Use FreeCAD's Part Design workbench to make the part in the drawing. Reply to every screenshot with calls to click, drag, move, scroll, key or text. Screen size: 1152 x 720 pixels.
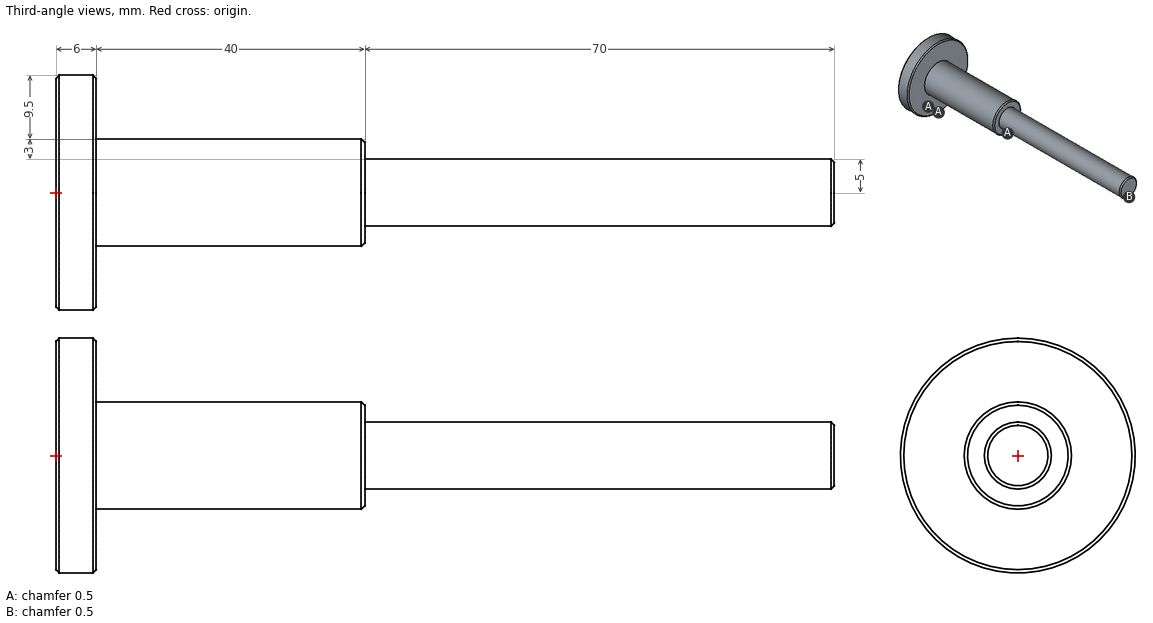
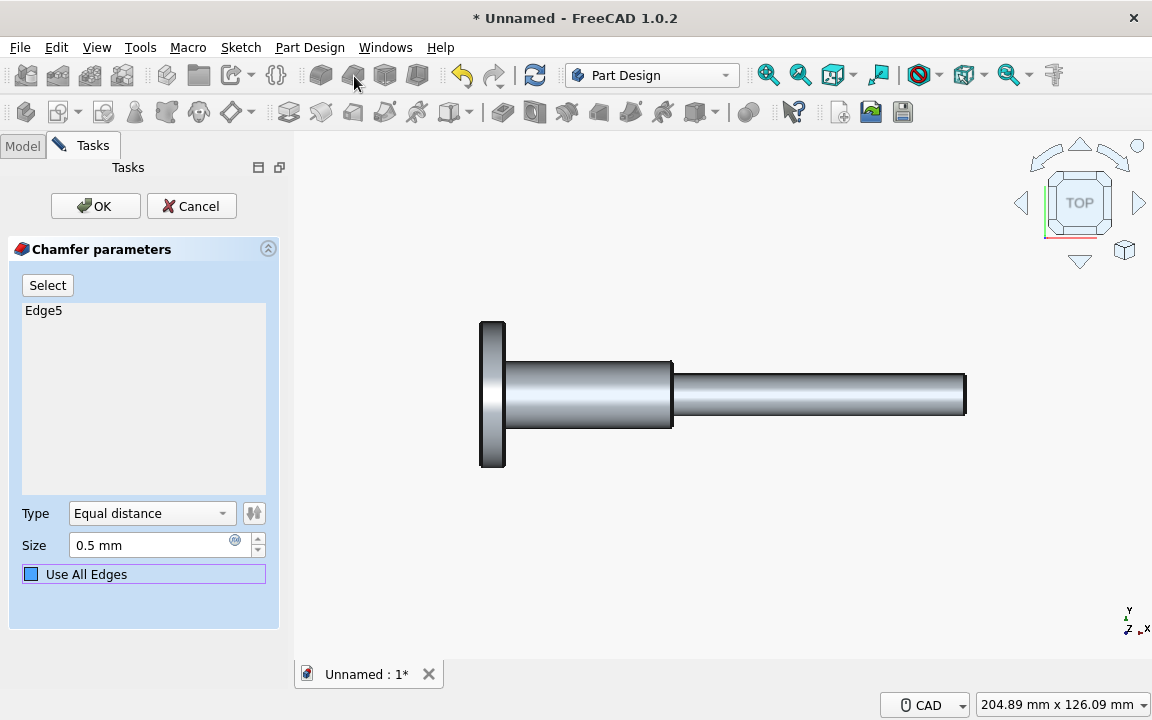
click(96, 206)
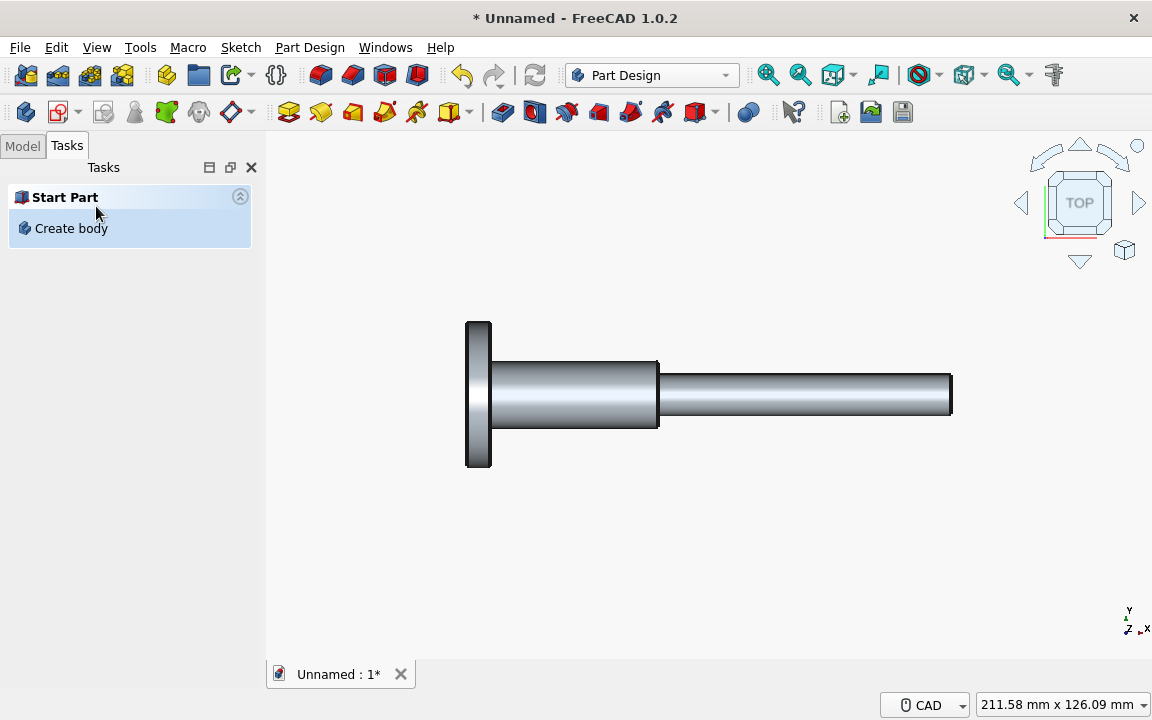
key(0)